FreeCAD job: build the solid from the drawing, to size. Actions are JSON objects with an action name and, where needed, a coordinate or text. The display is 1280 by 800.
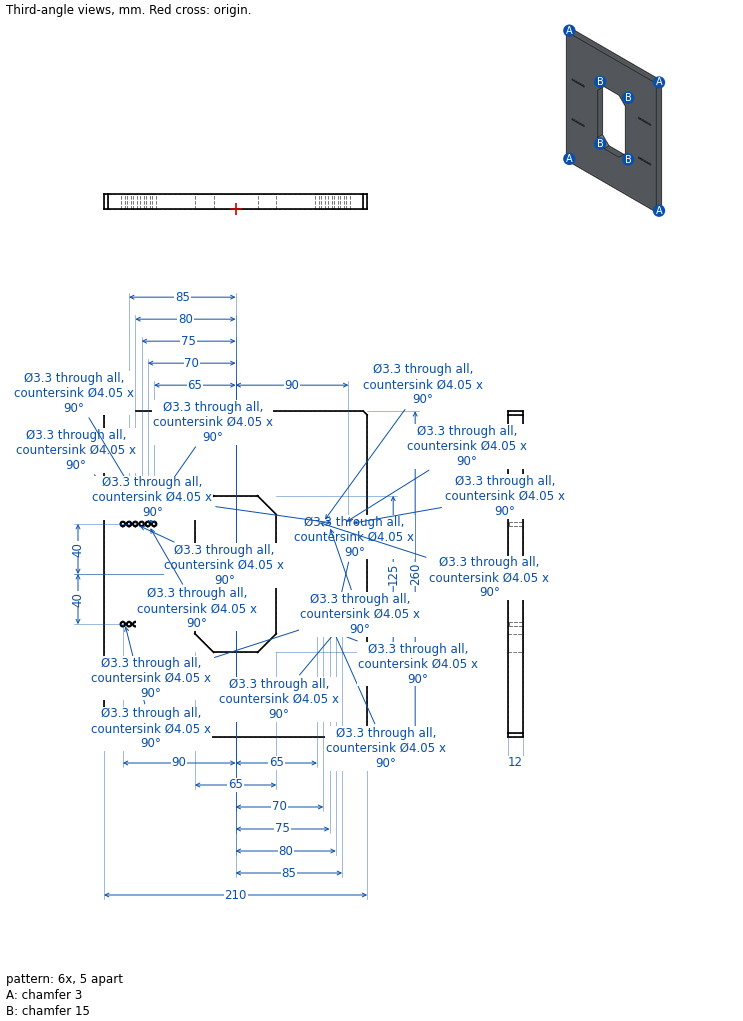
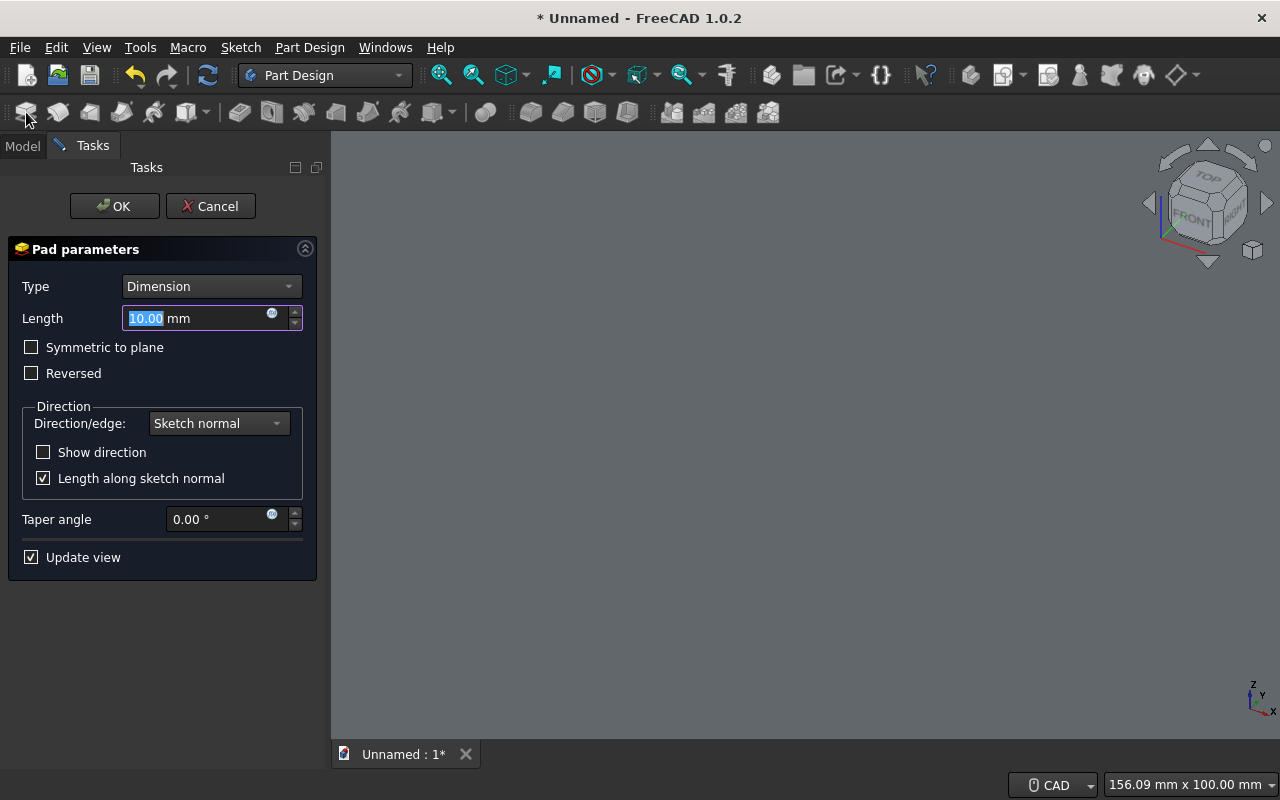
{"action": "type", "text": "12"}
{"action": "key", "text": "Tab"}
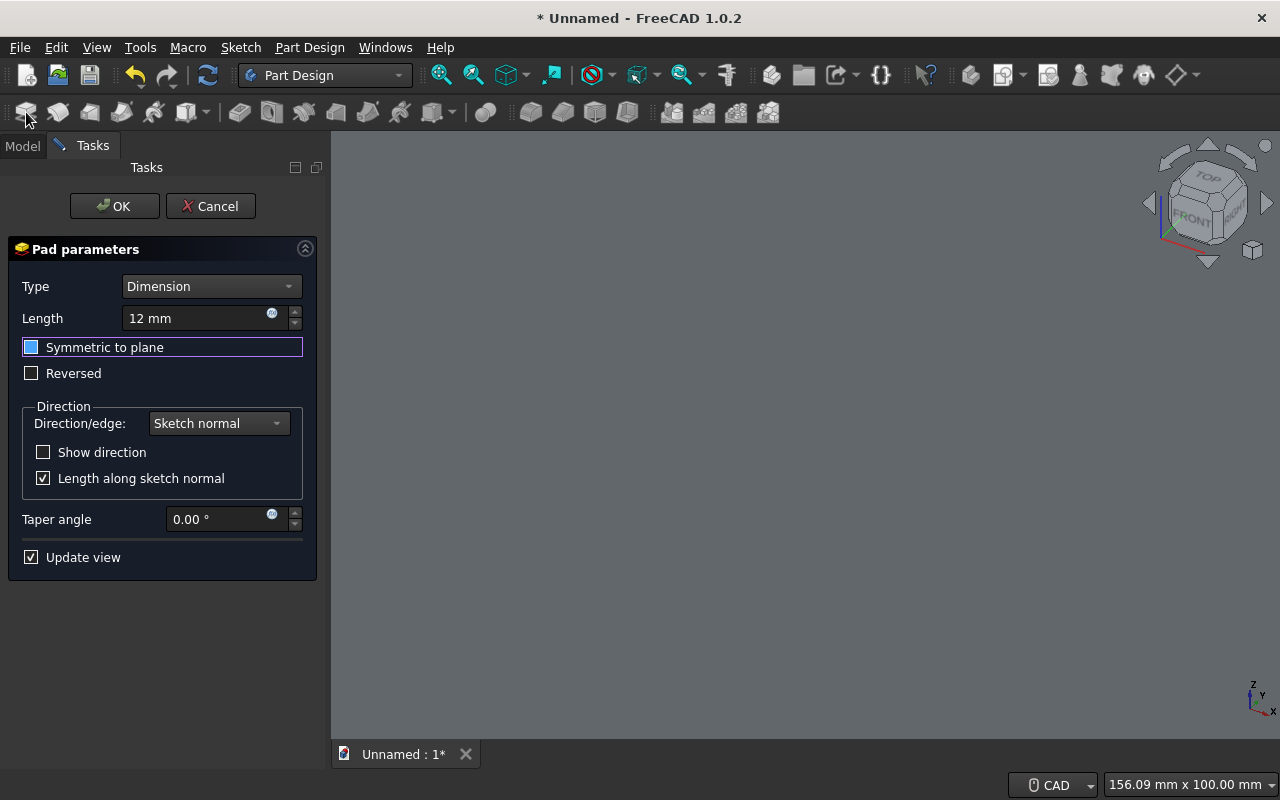
{"action": "left_click", "coordinate": [30, 373]}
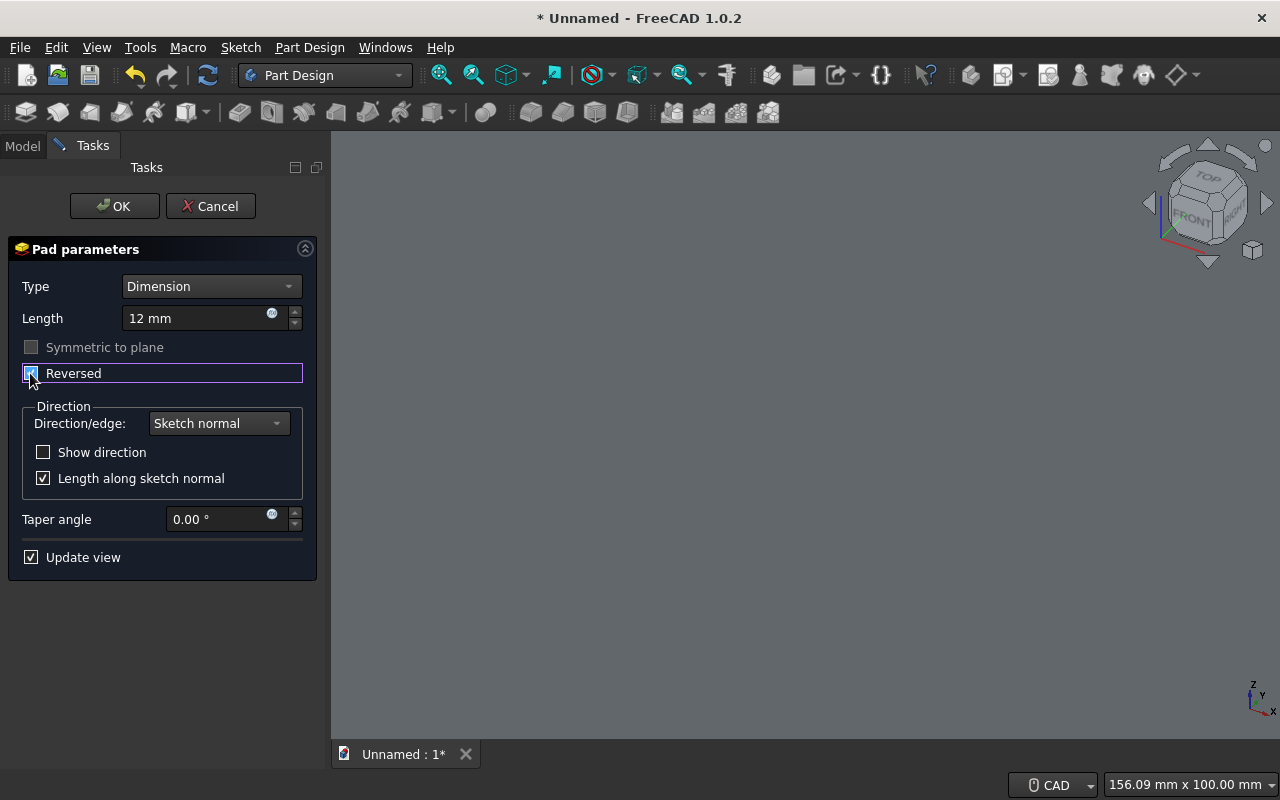
{"action": "left_click", "coordinate": [115, 206]}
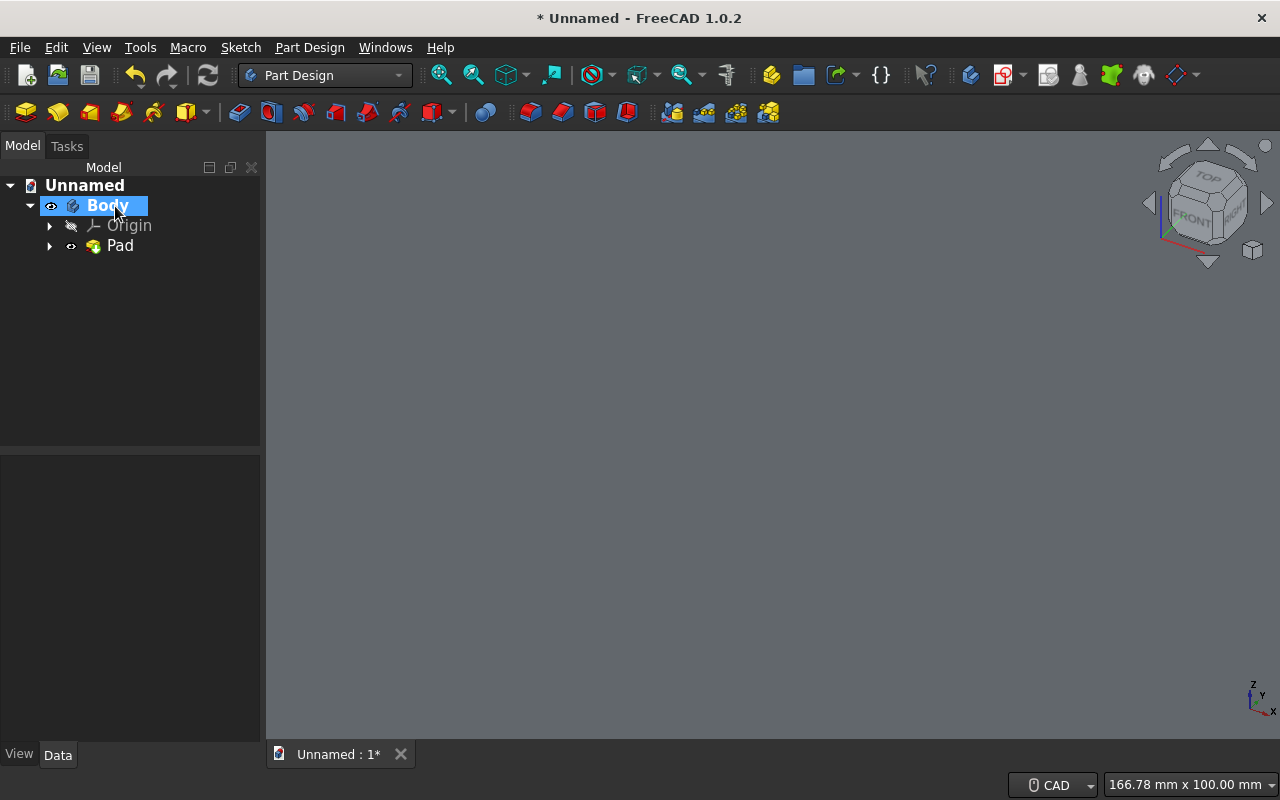
{"action": "left_click", "coordinate": [442, 76]}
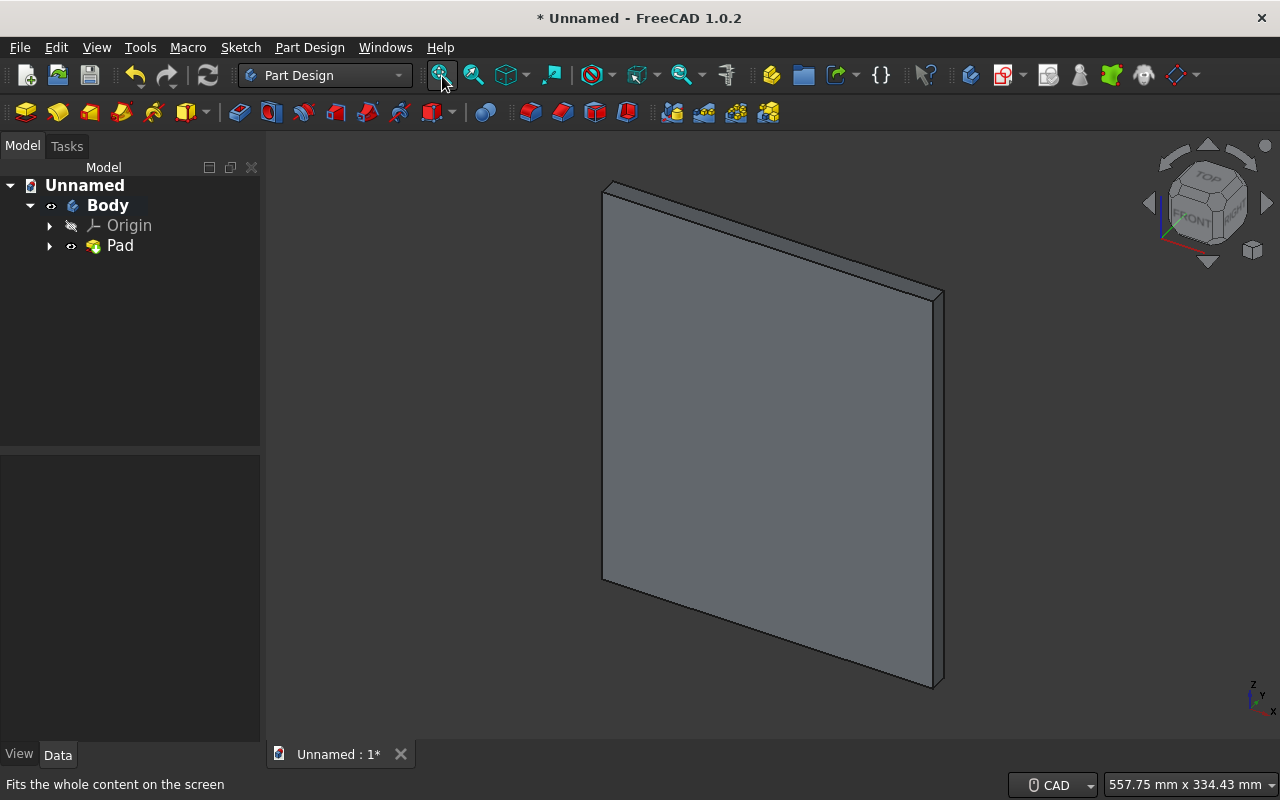
{"action": "left_click", "coordinate": [1004, 76]}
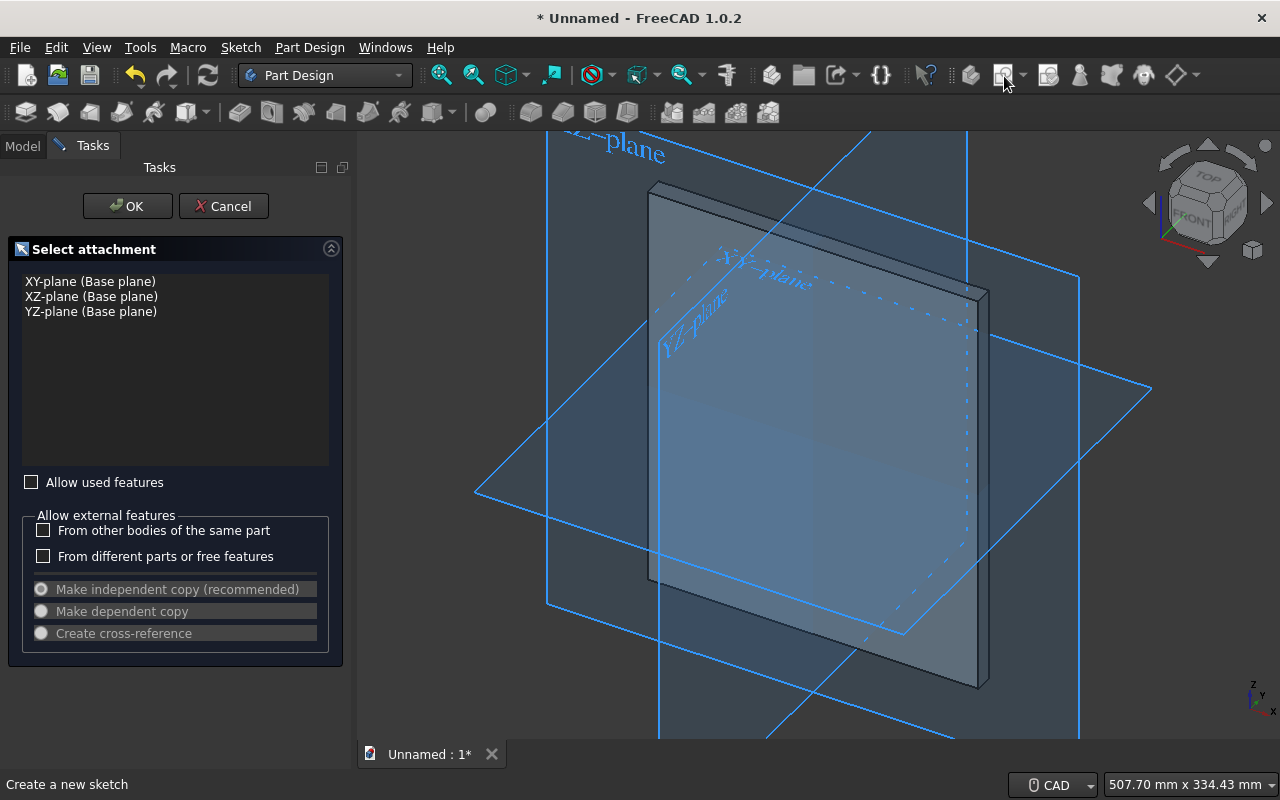
{"action": "left_click", "coordinate": [82, 296]}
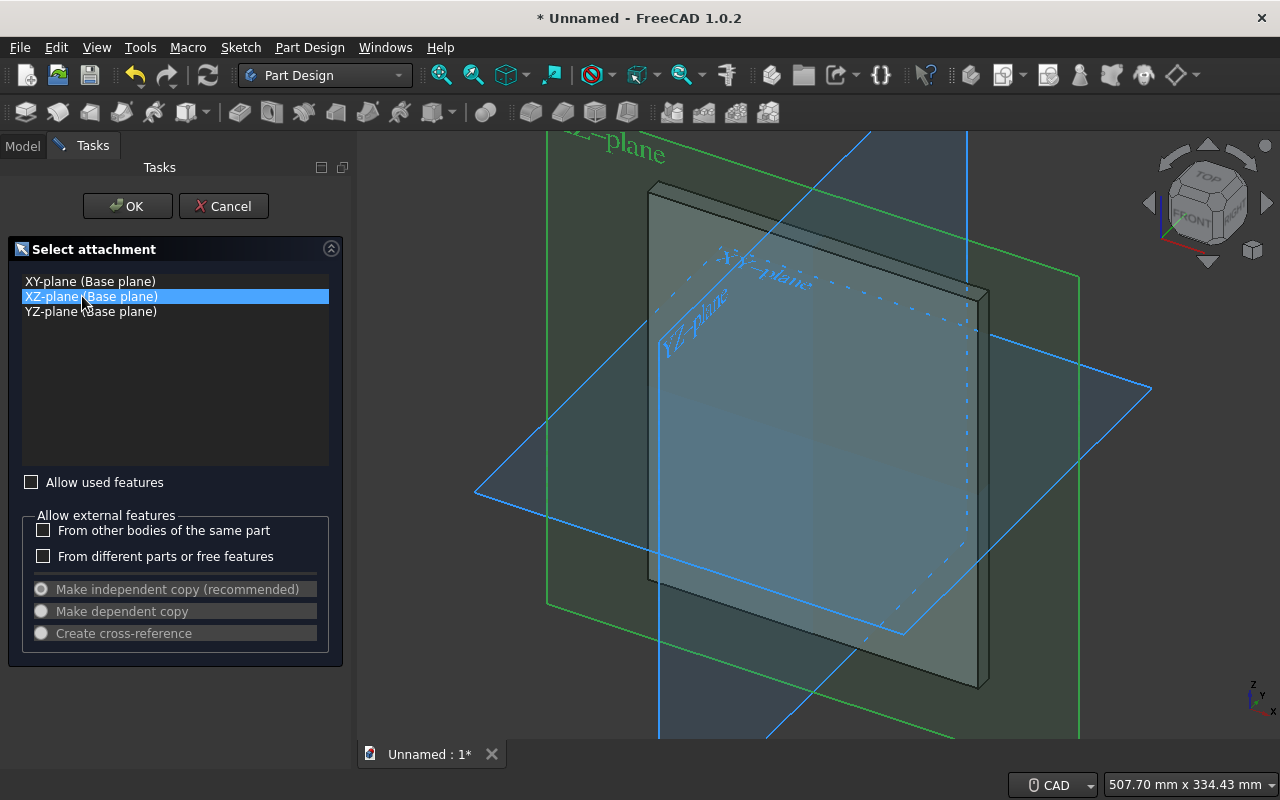
{"action": "left_click", "coordinate": [128, 206]}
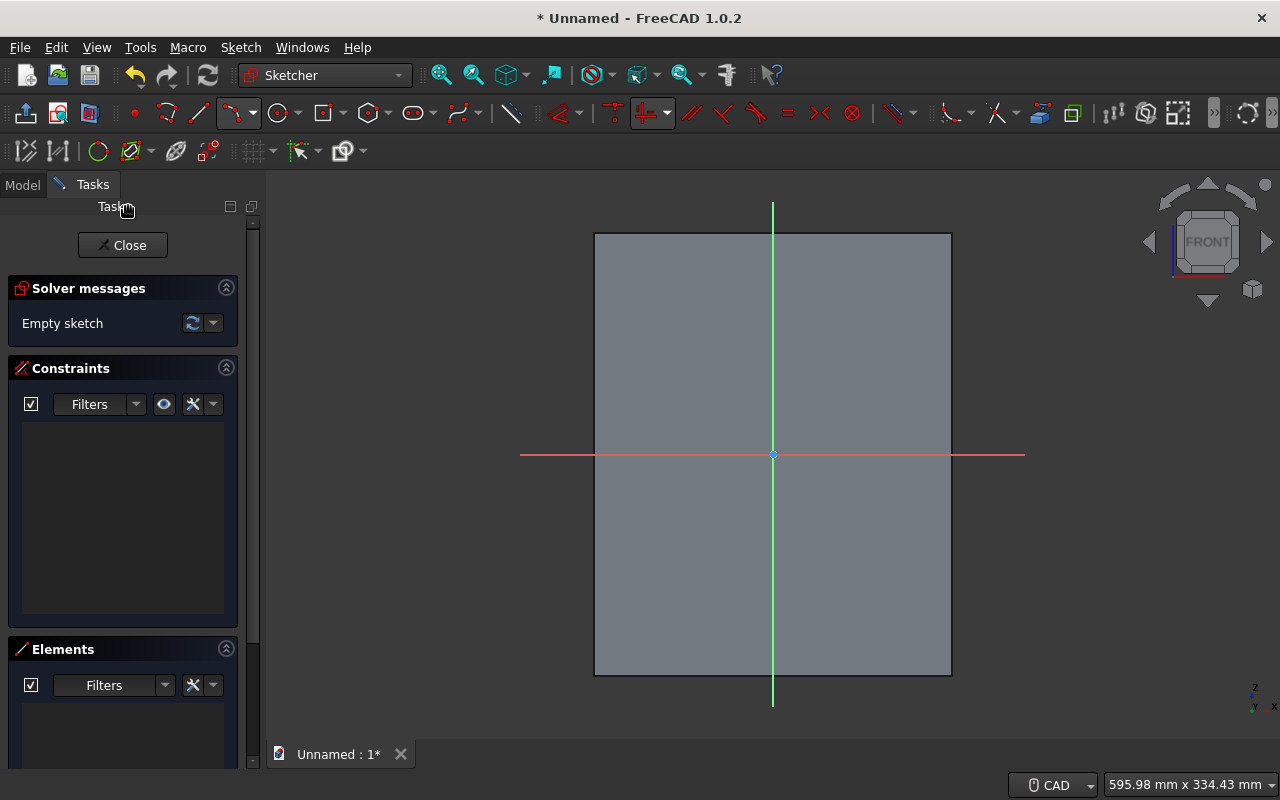
{"action": "scroll", "coordinate": [615, 526], "scroll_direction": "up", "scroll_amount": 15}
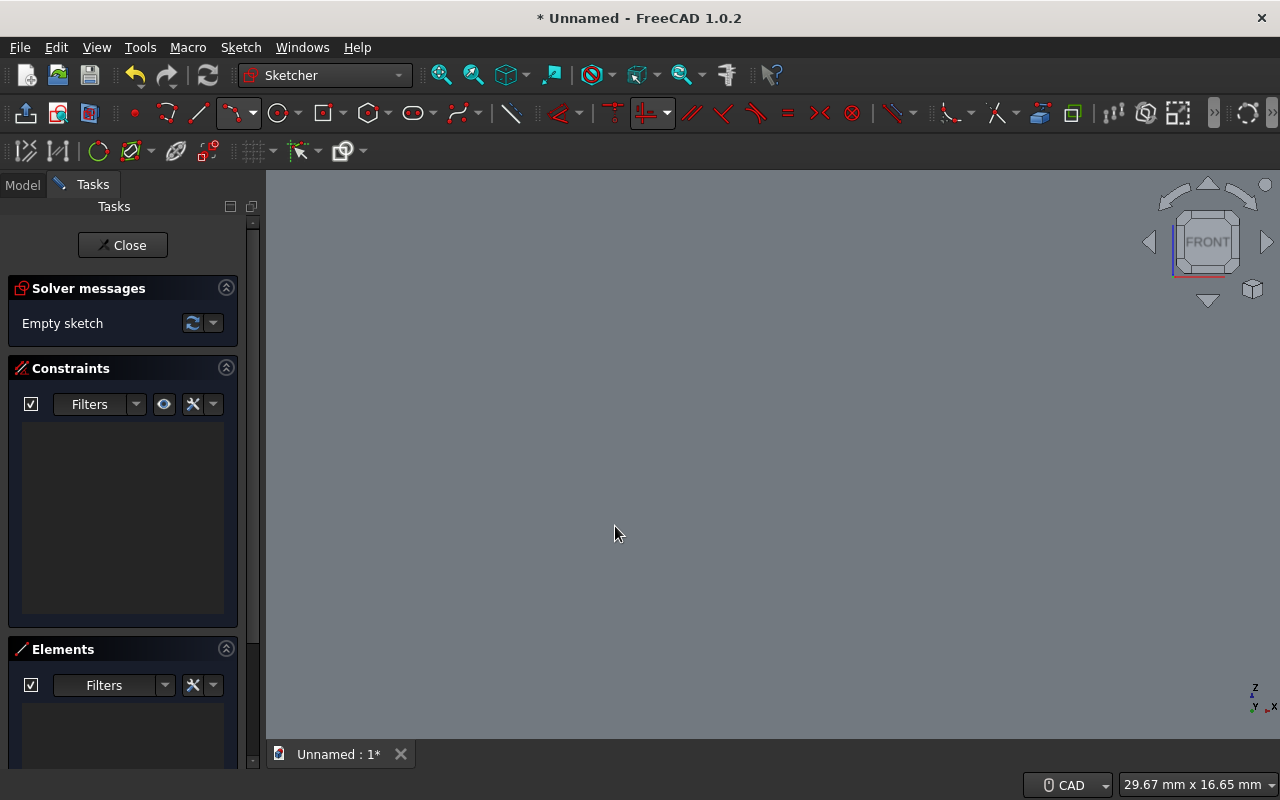
{"action": "scroll", "coordinate": [707, 441], "scroll_direction": "up", "scroll_amount": 6}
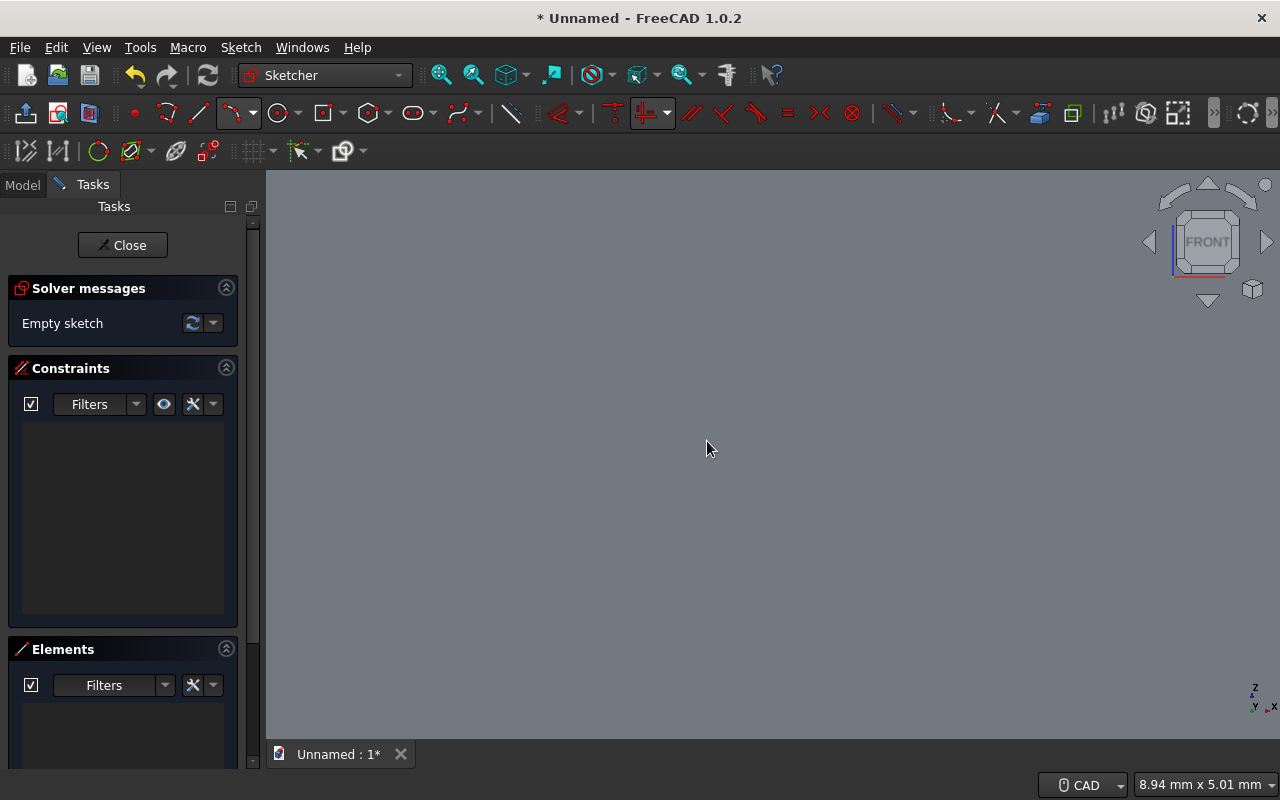
{"action": "left_click", "coordinate": [278, 114]}